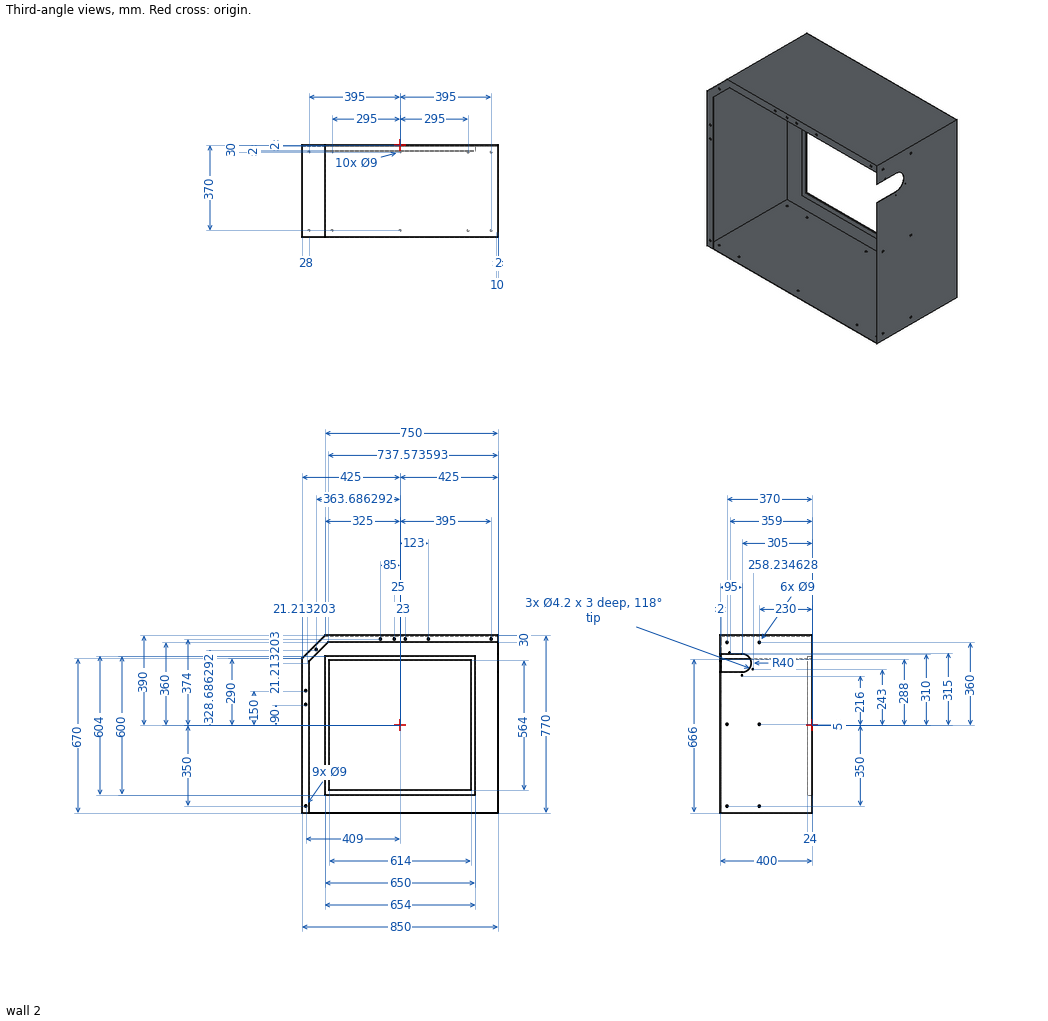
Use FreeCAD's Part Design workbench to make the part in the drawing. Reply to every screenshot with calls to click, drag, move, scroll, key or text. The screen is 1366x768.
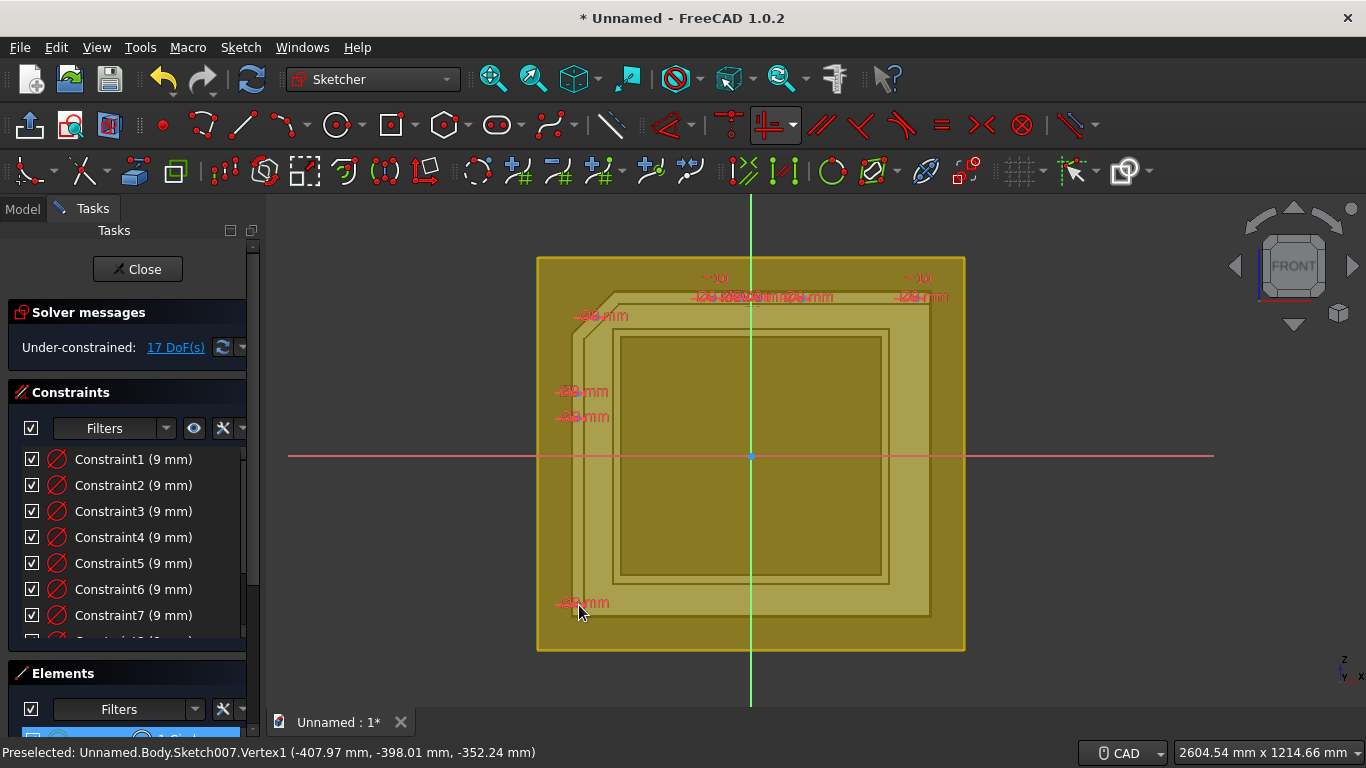
click(579, 419)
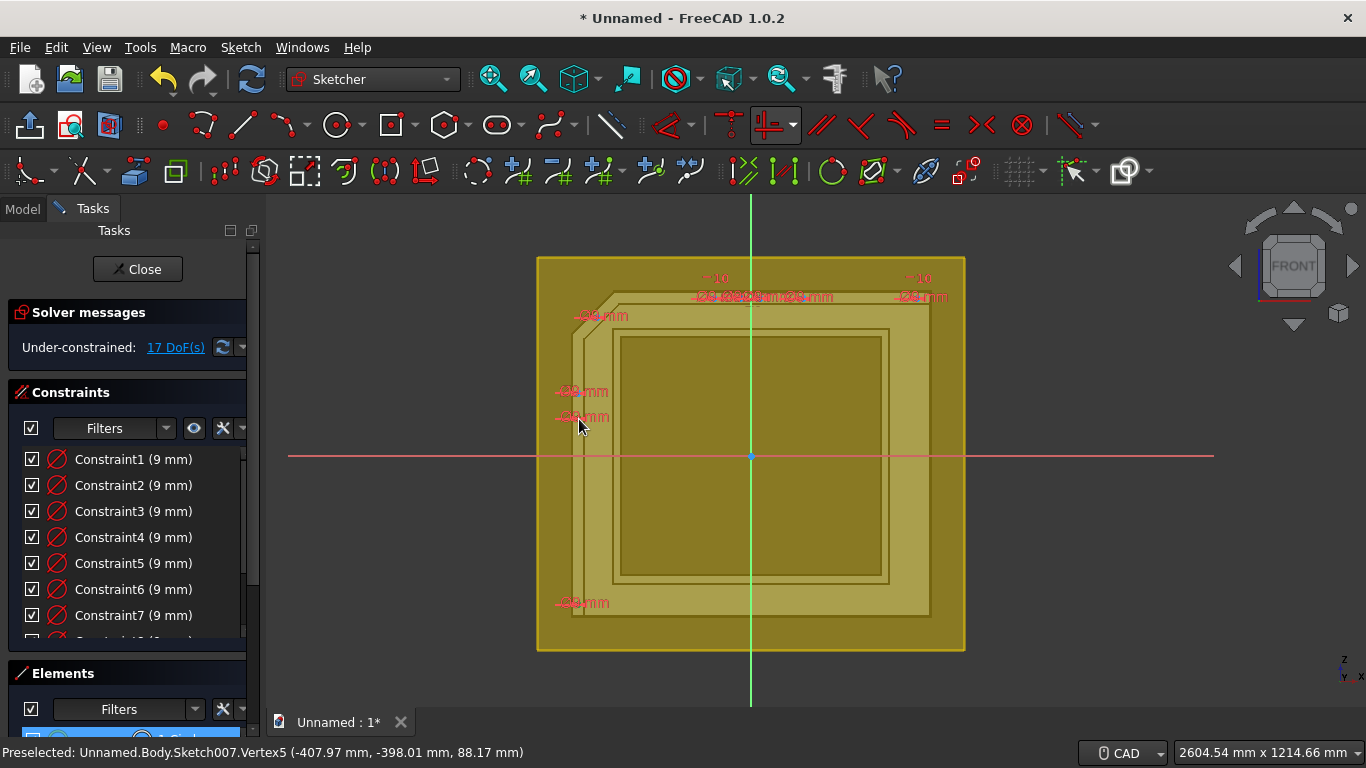
key(v)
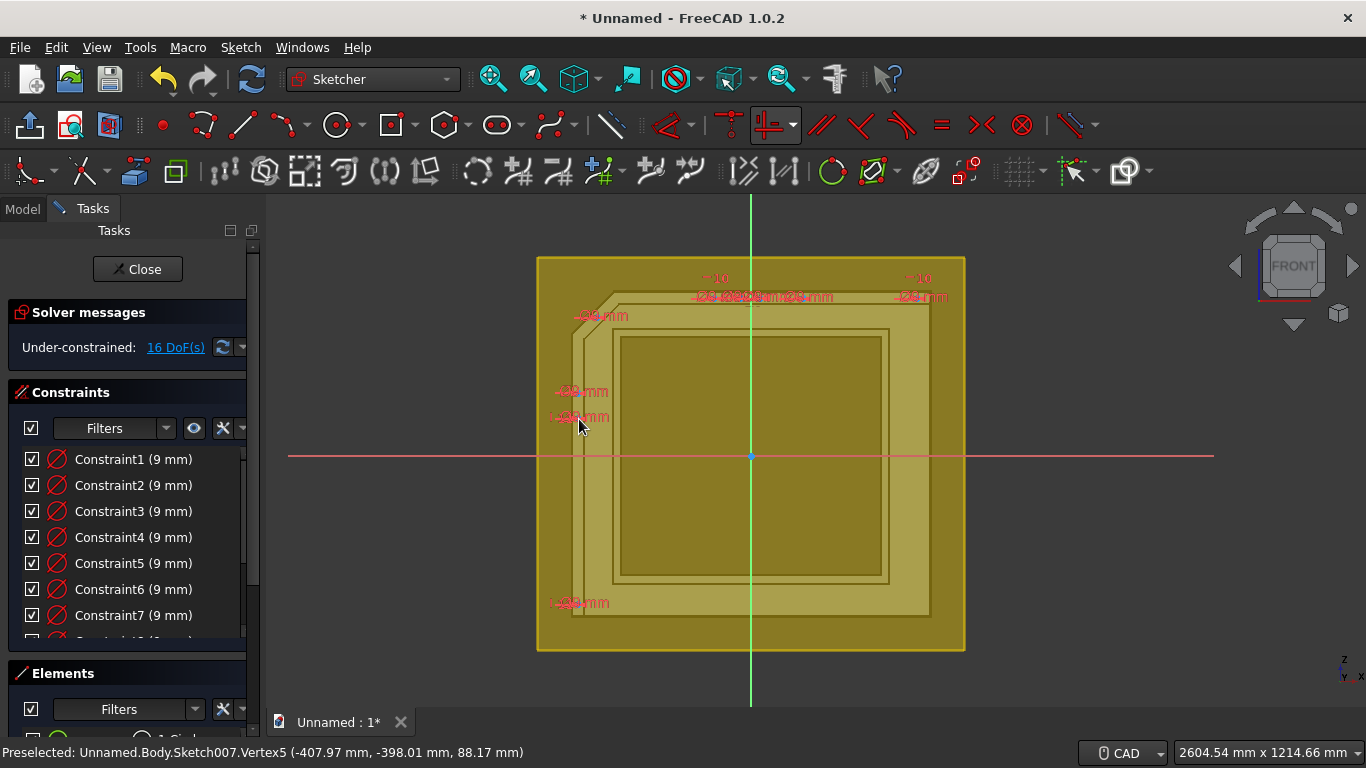
click(715, 299)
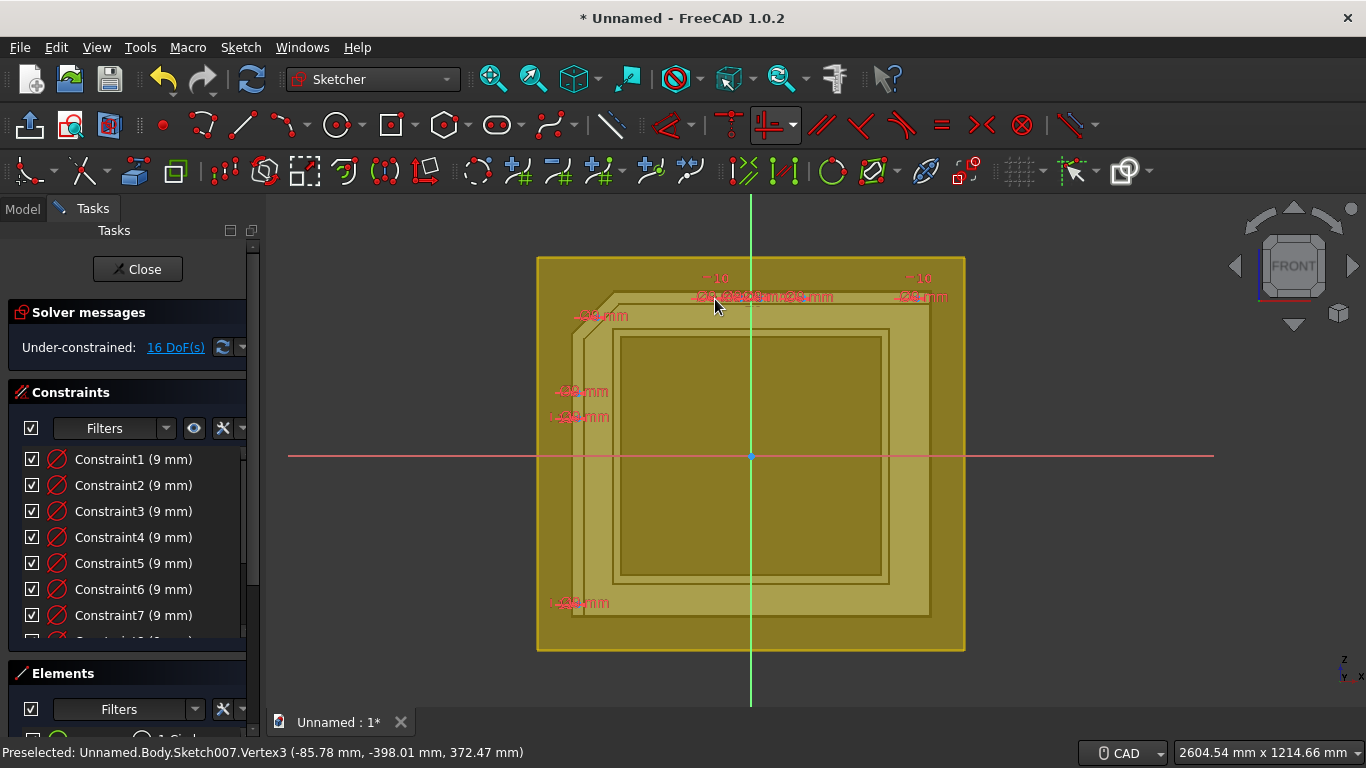
click(740, 298)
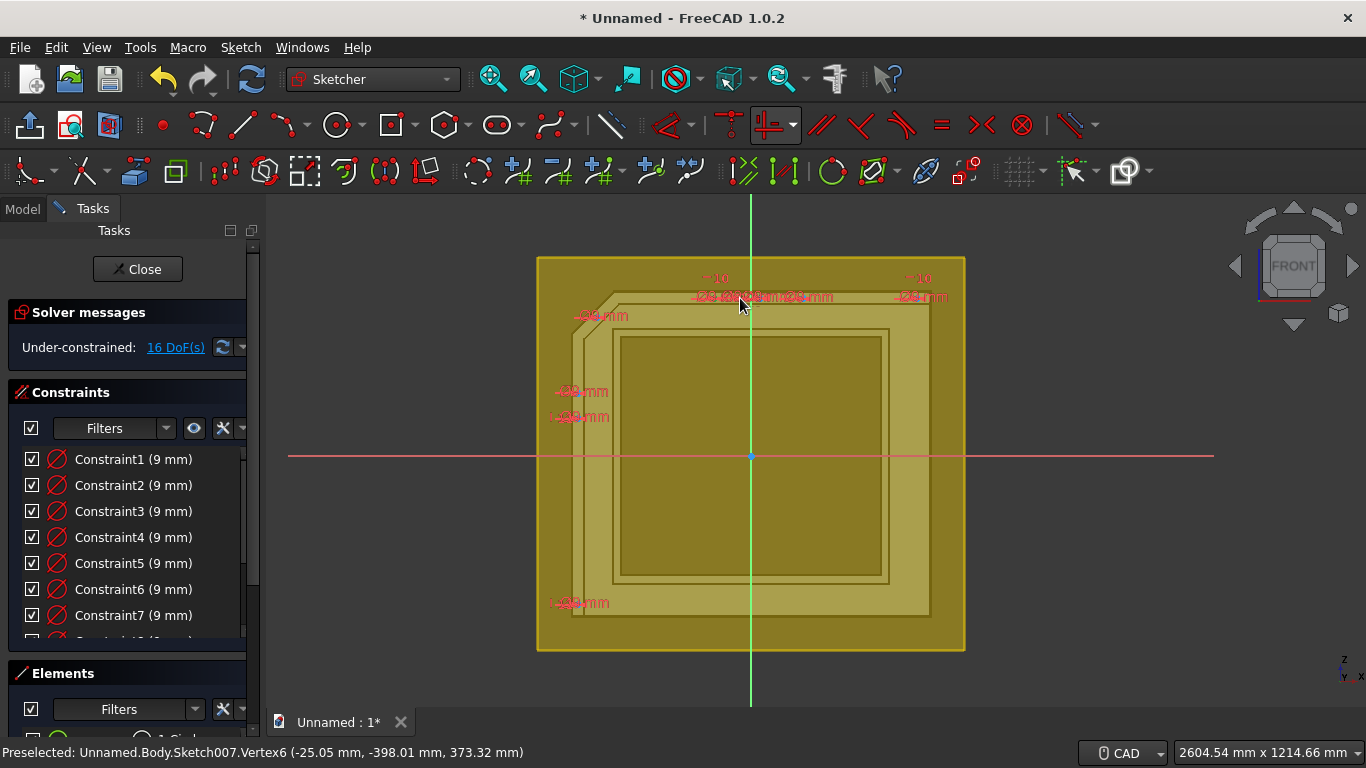
click(796, 126)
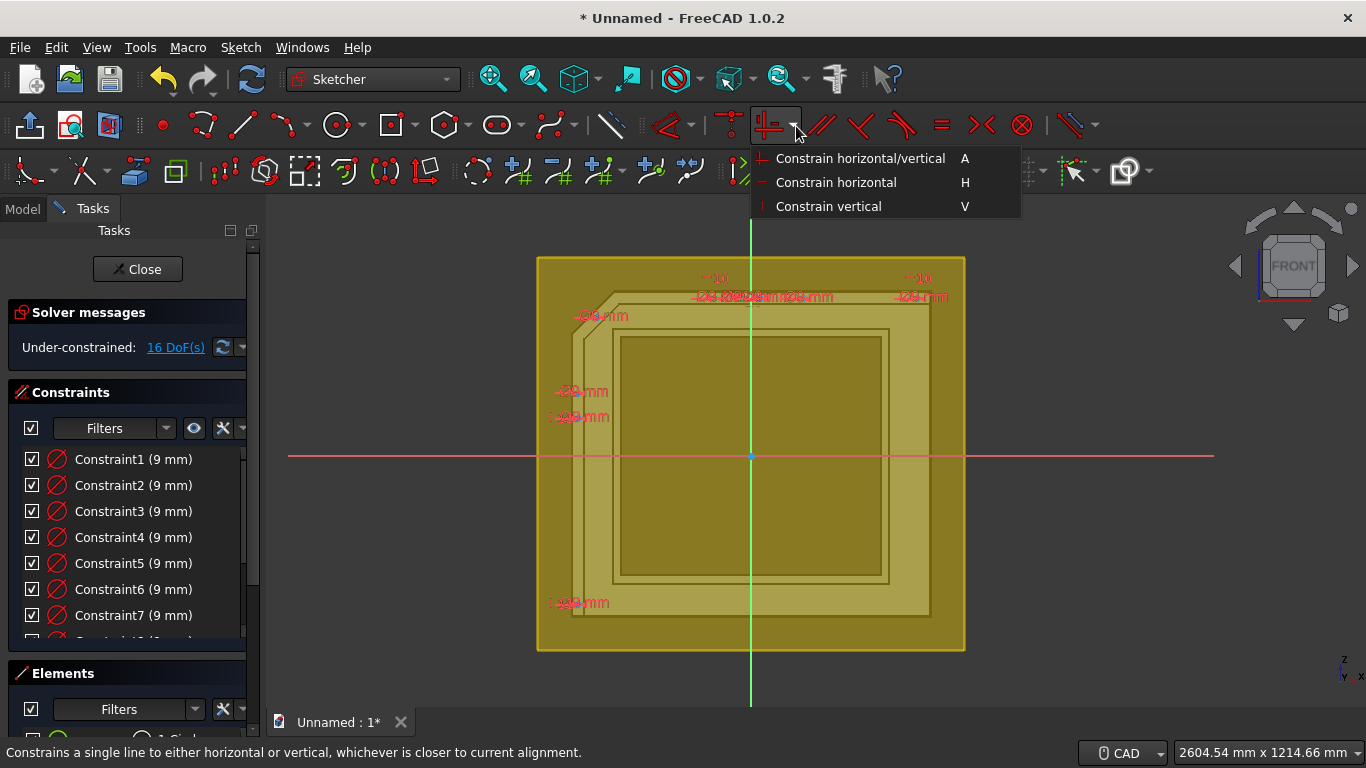
click(886, 182)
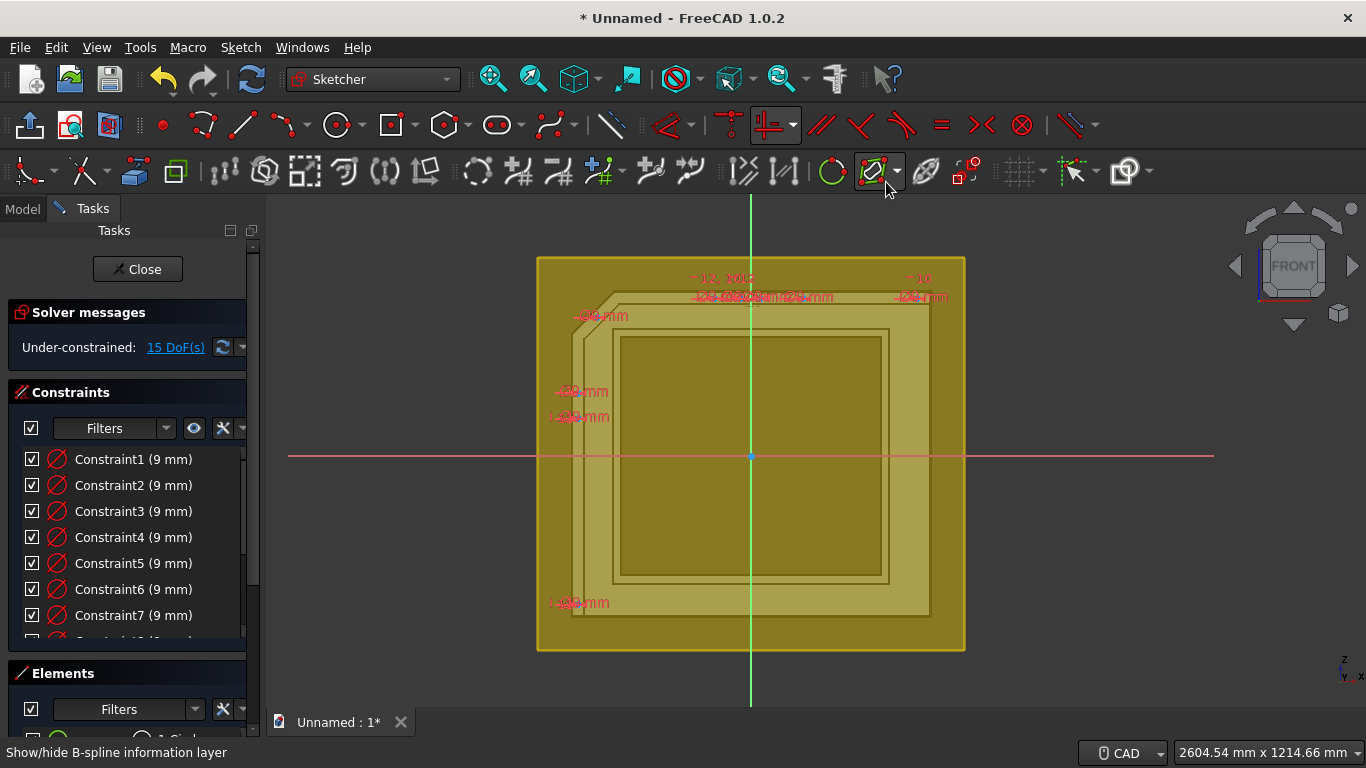
click(579, 419)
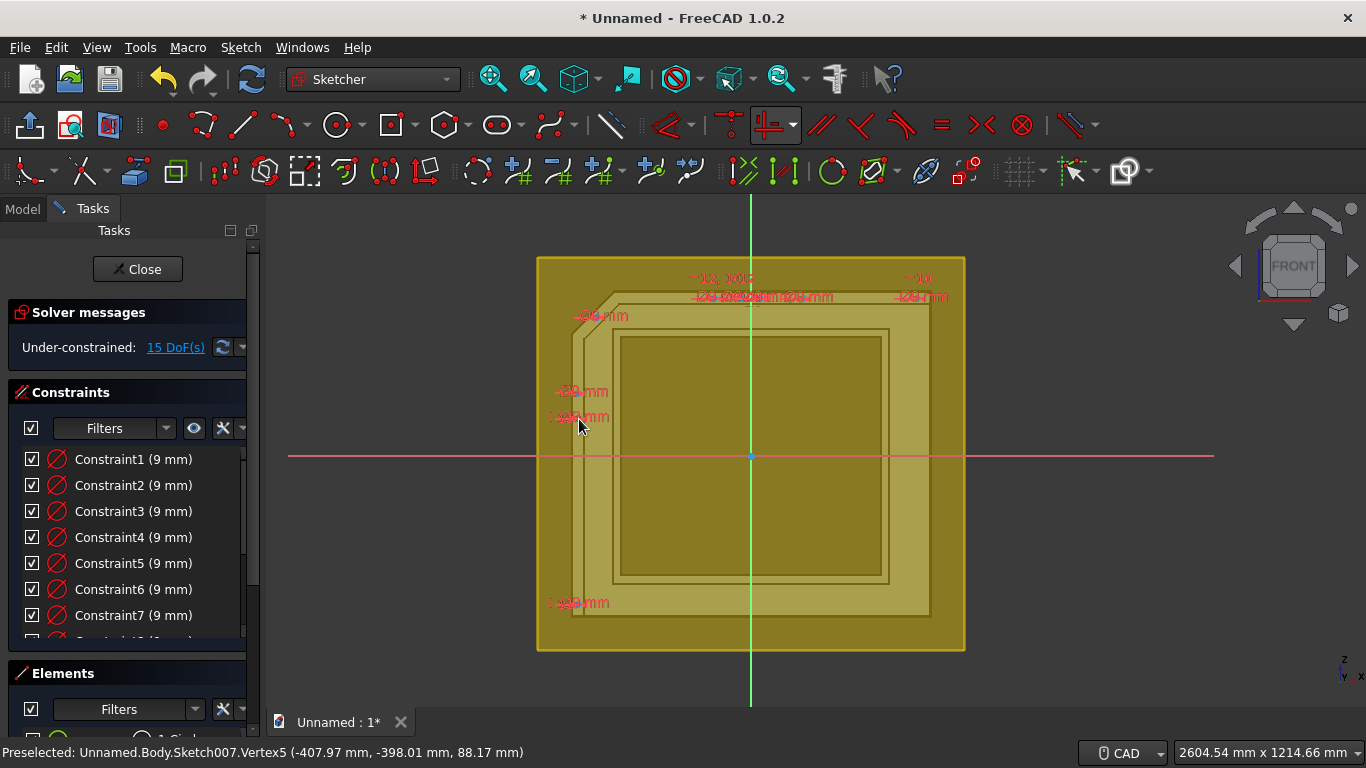
click(578, 393)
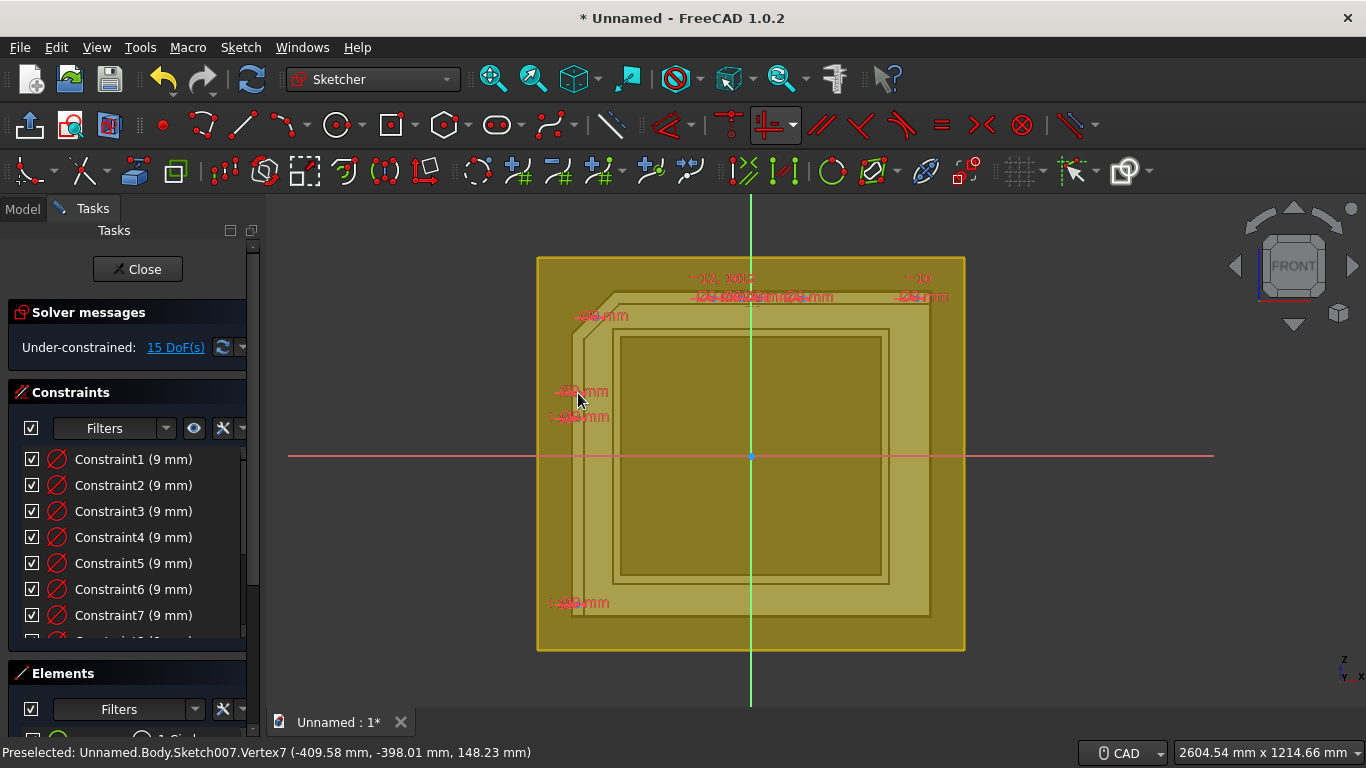
key(v)